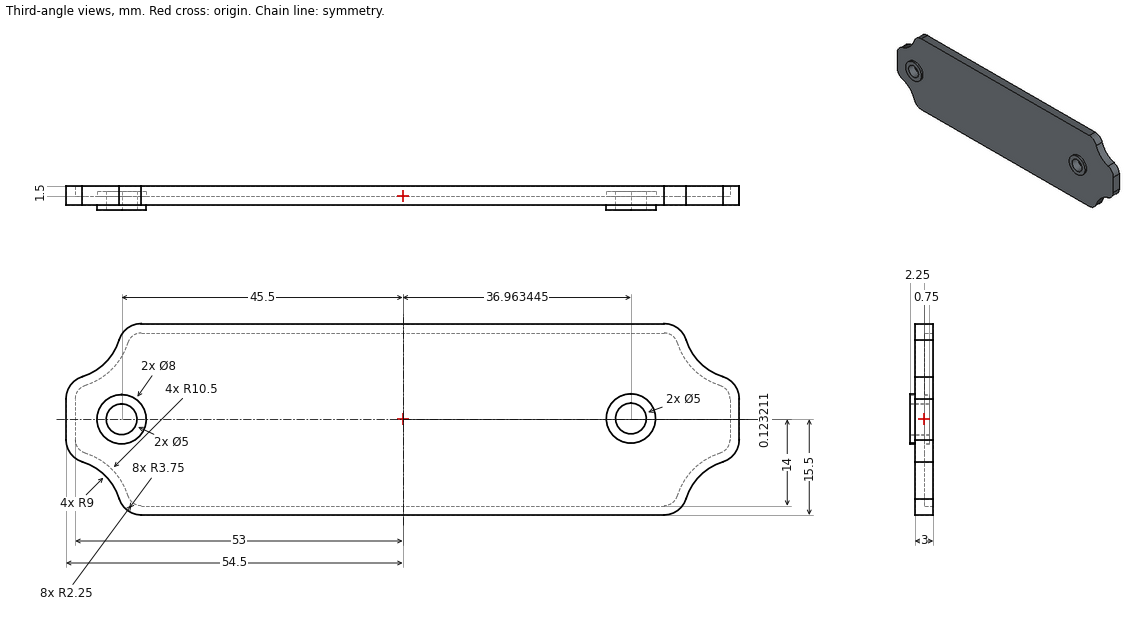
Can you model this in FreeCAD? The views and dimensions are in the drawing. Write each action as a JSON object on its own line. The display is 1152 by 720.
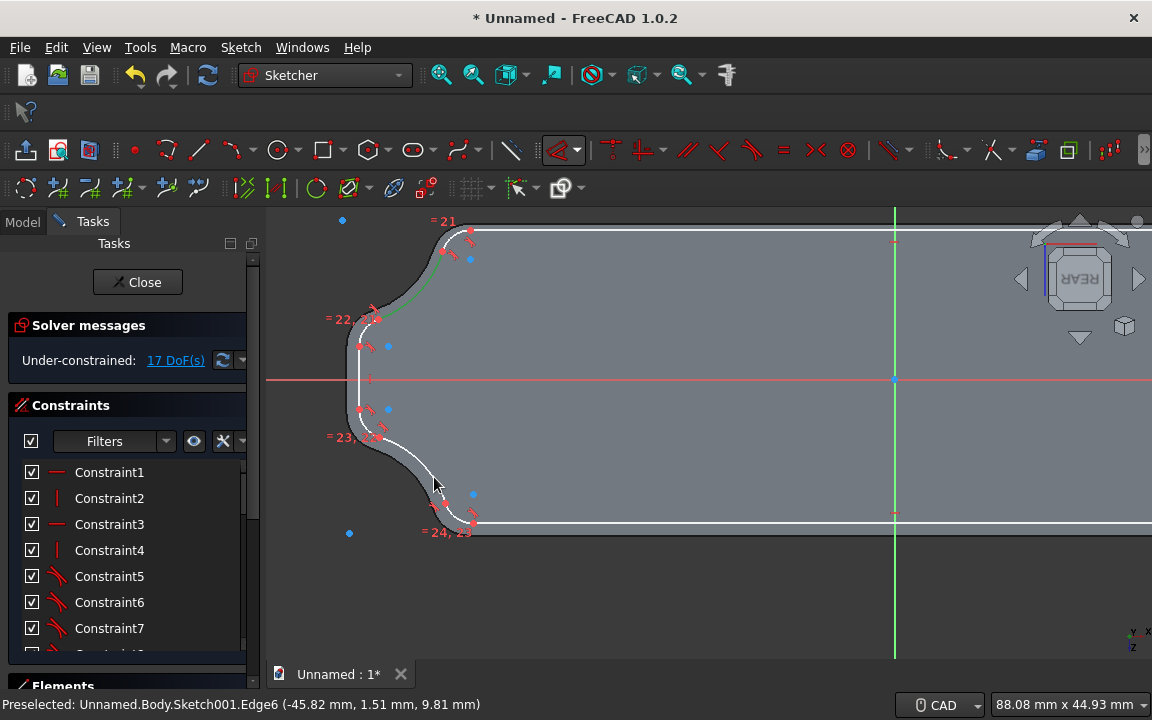
{"action": "left_click", "coordinate": [433, 477]}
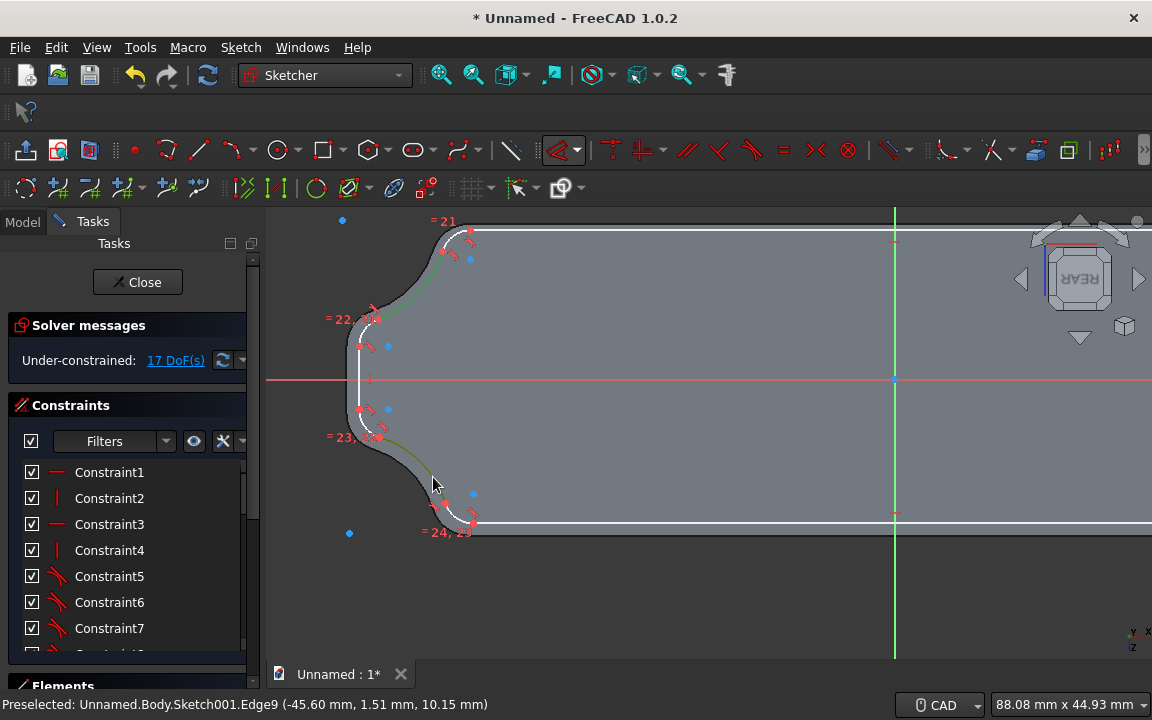
{"action": "scroll", "coordinate": [433, 476], "scroll_direction": "down", "scroll_amount": 4}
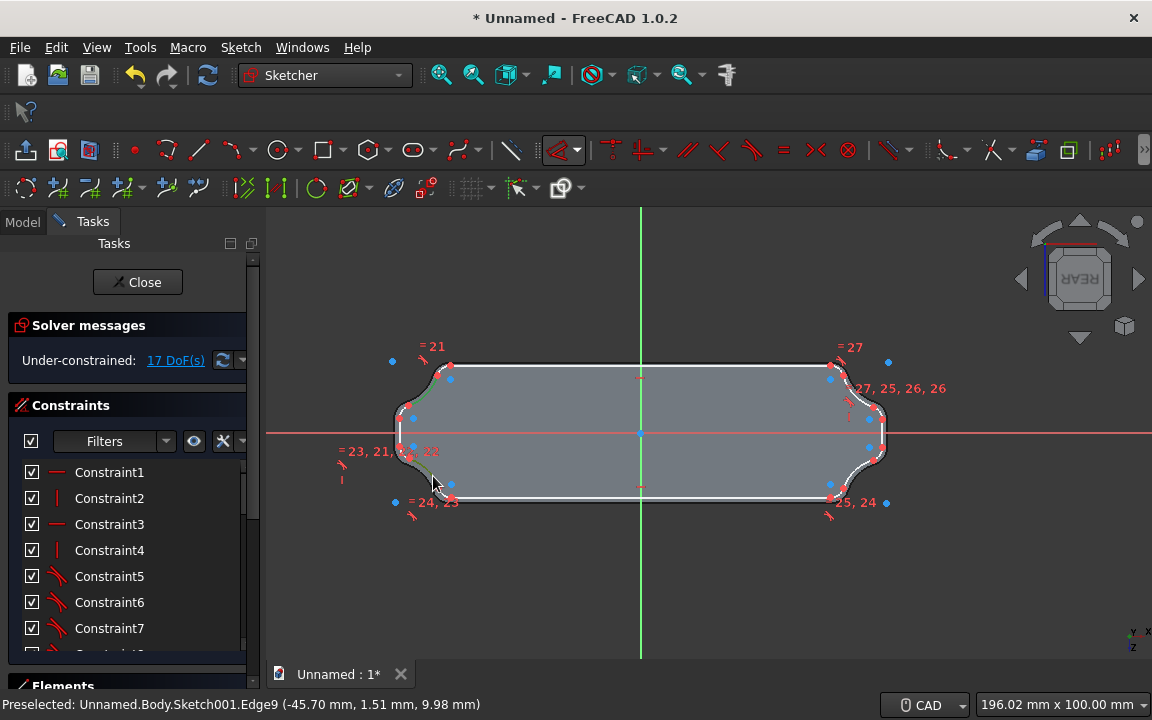
{"action": "left_click", "coordinate": [861, 465]}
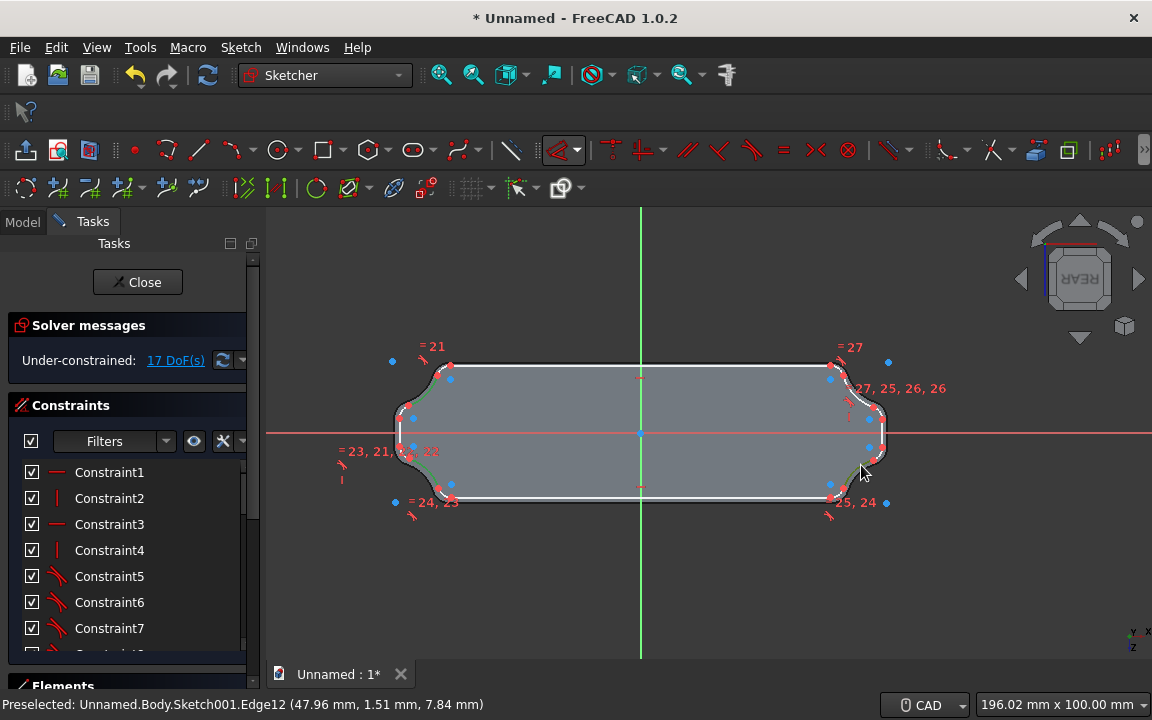
{"action": "scroll", "coordinate": [849, 388], "scroll_direction": "up", "scroll_amount": 4}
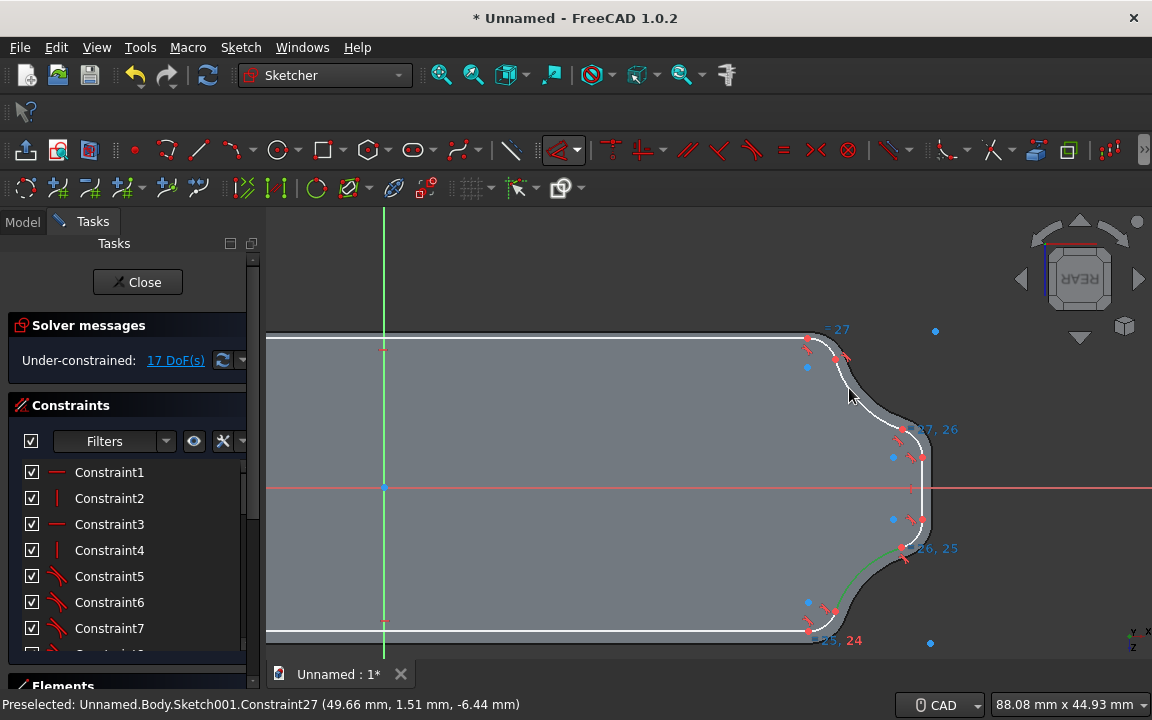
{"action": "left_click", "coordinate": [848, 387]}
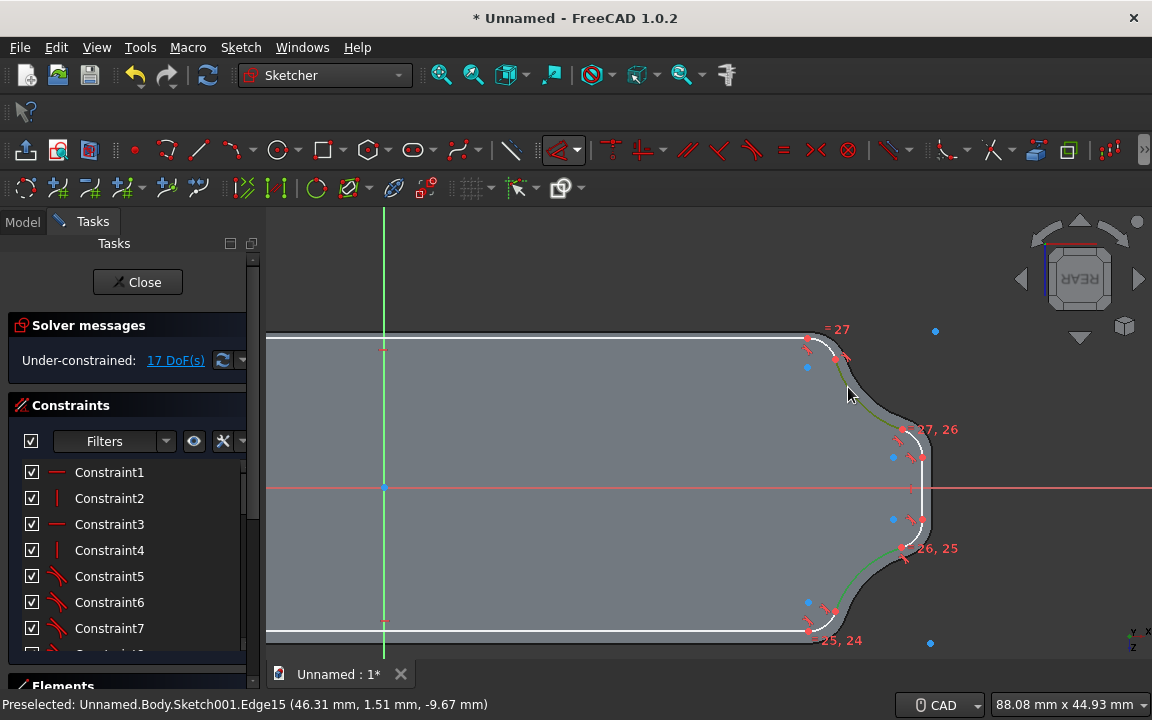
{"action": "left_click", "coordinate": [784, 150]}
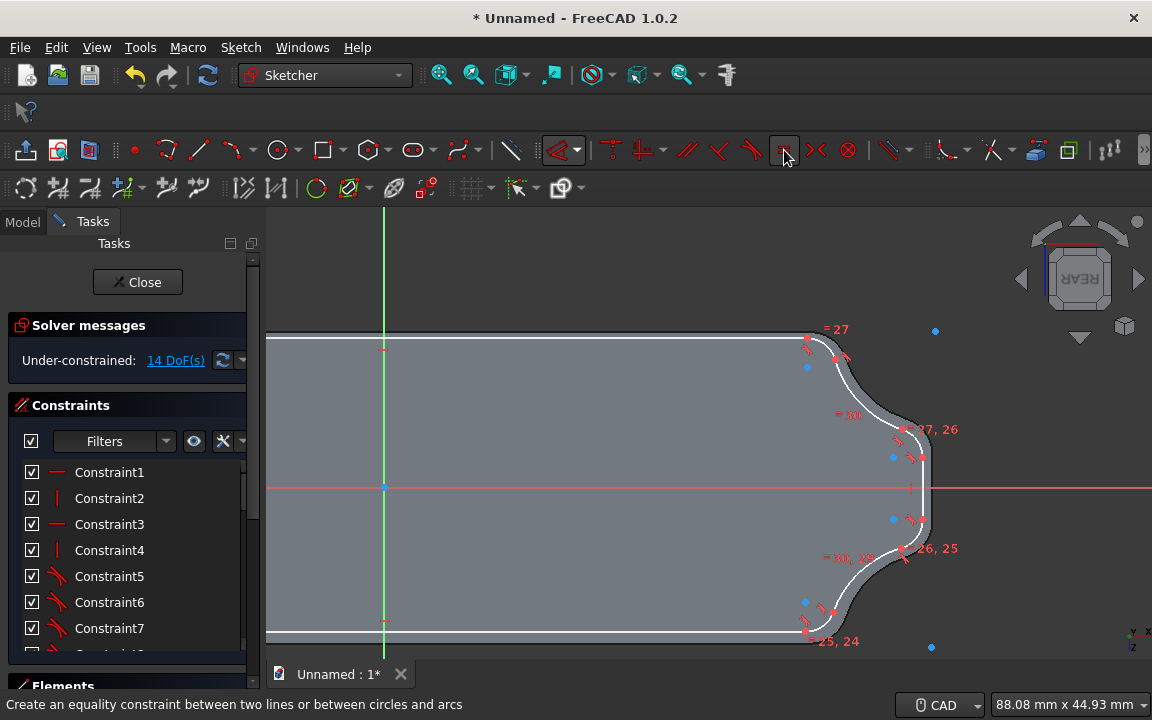
{"action": "scroll", "coordinate": [850, 388], "scroll_direction": "down", "scroll_amount": 4}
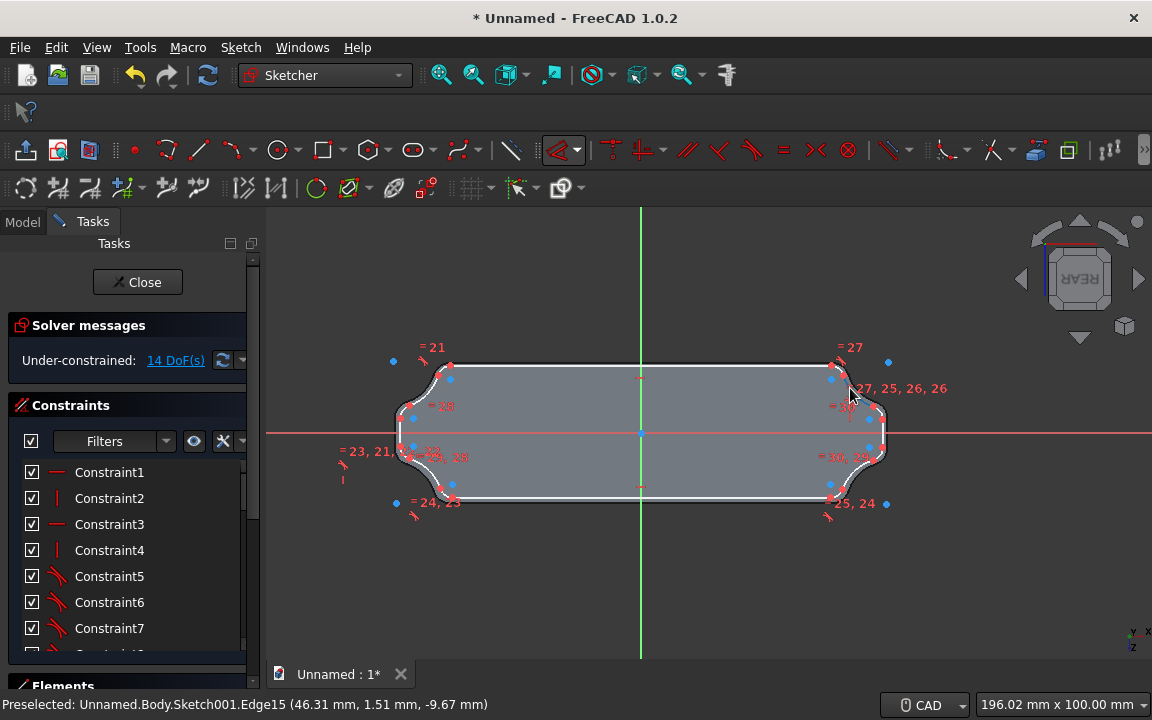
{"action": "left_click", "coordinate": [393, 362]}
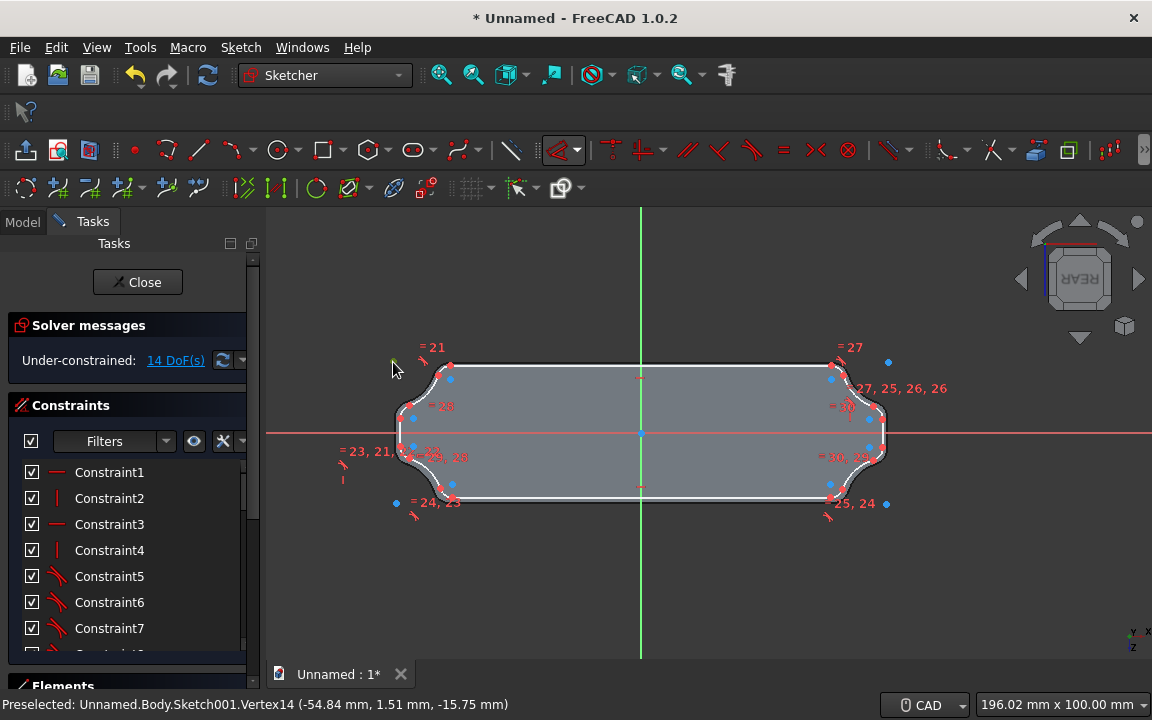
{"action": "left_click", "coordinate": [396, 504]}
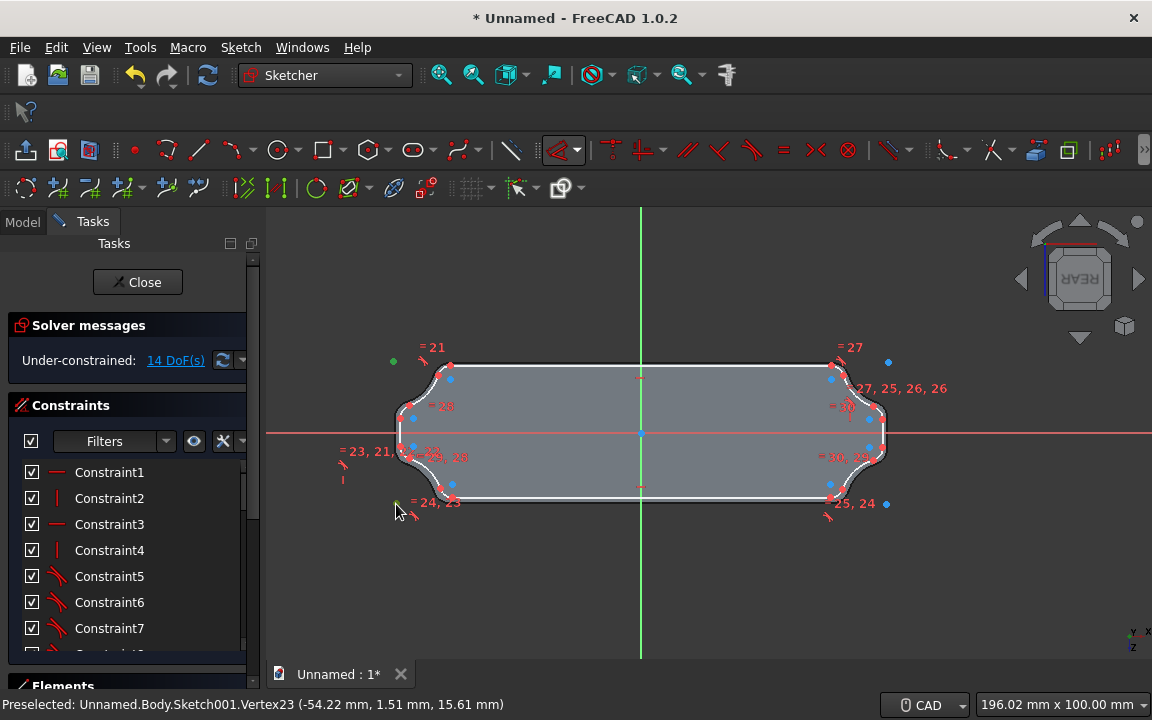
{"action": "left_click", "coordinate": [344, 433]}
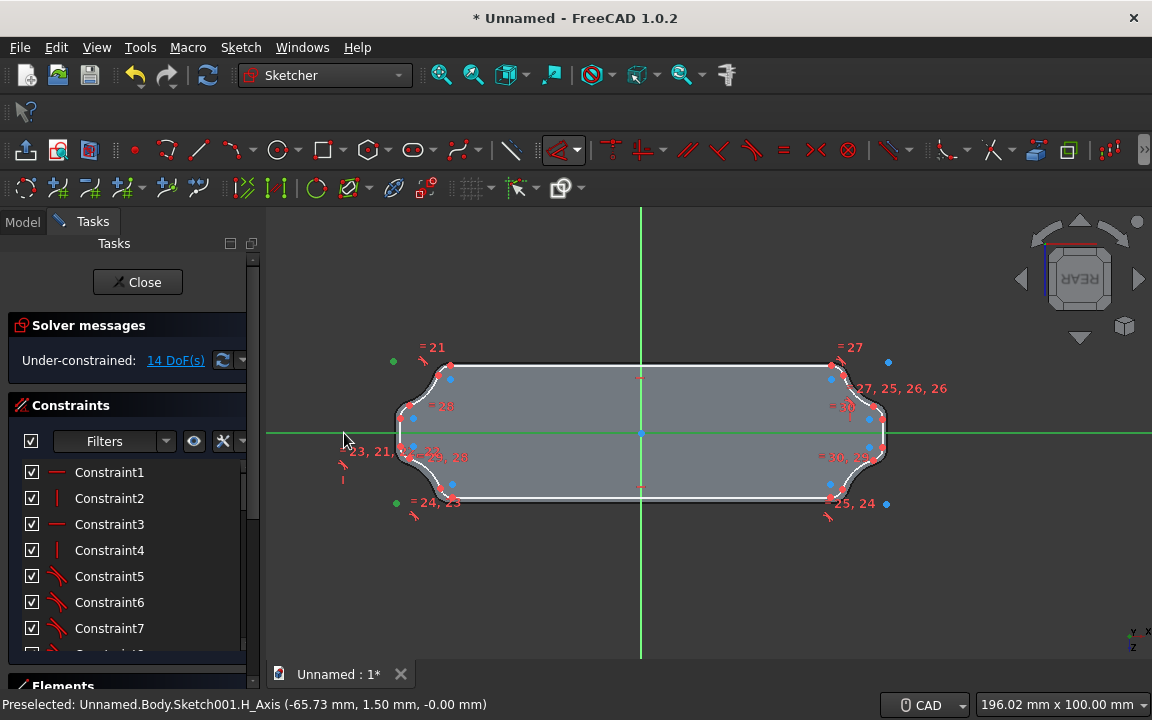
{"action": "left_click", "coordinate": [816, 150]}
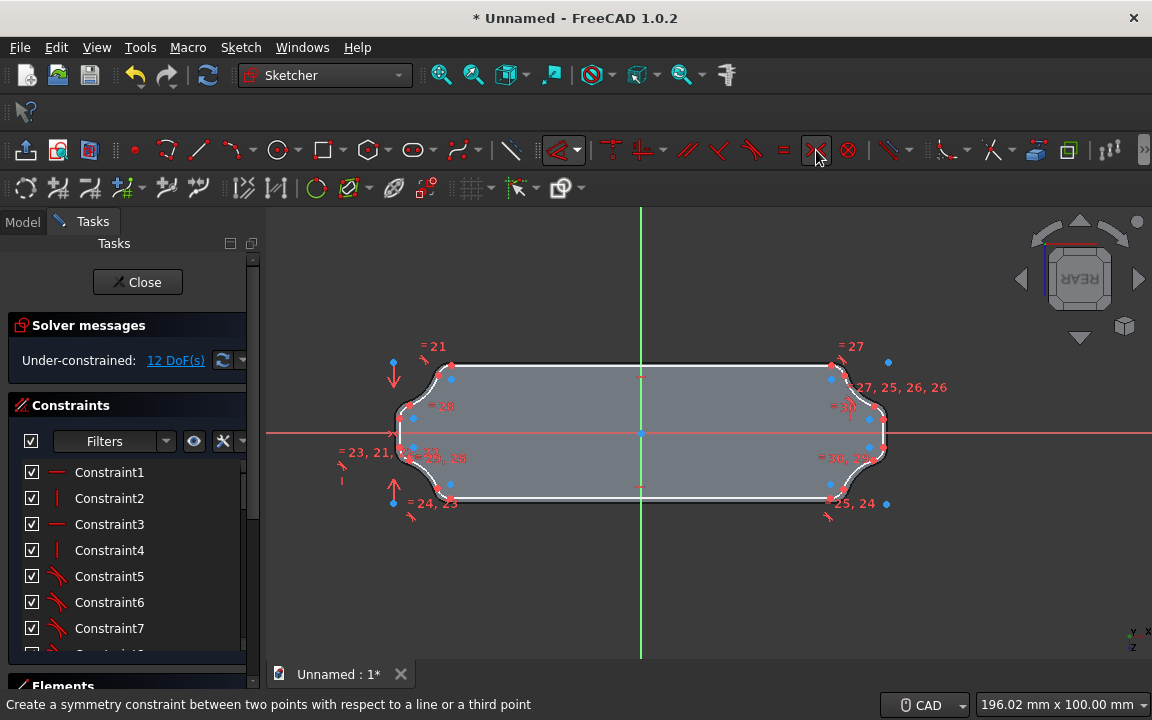
{"action": "left_click", "coordinate": [394, 504]}